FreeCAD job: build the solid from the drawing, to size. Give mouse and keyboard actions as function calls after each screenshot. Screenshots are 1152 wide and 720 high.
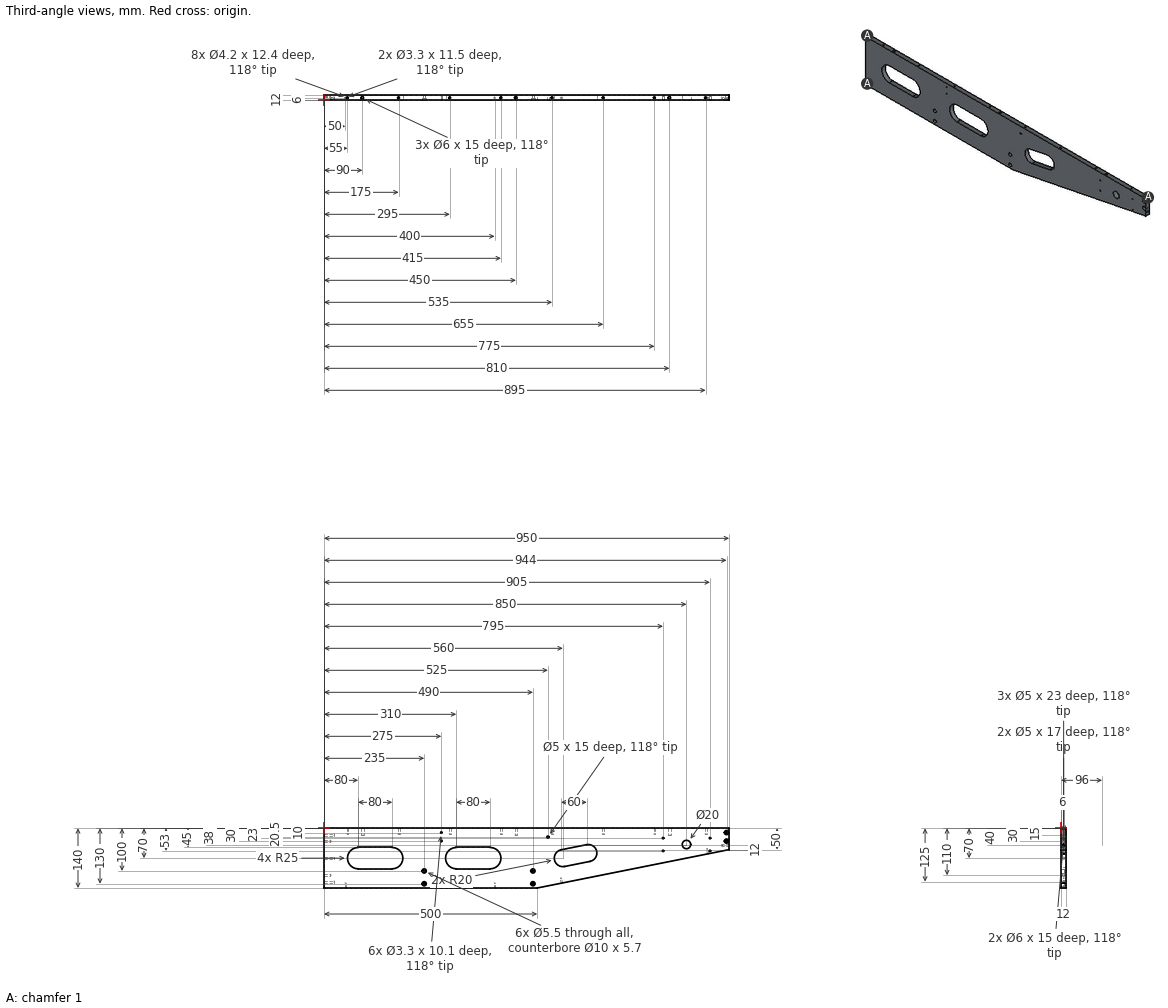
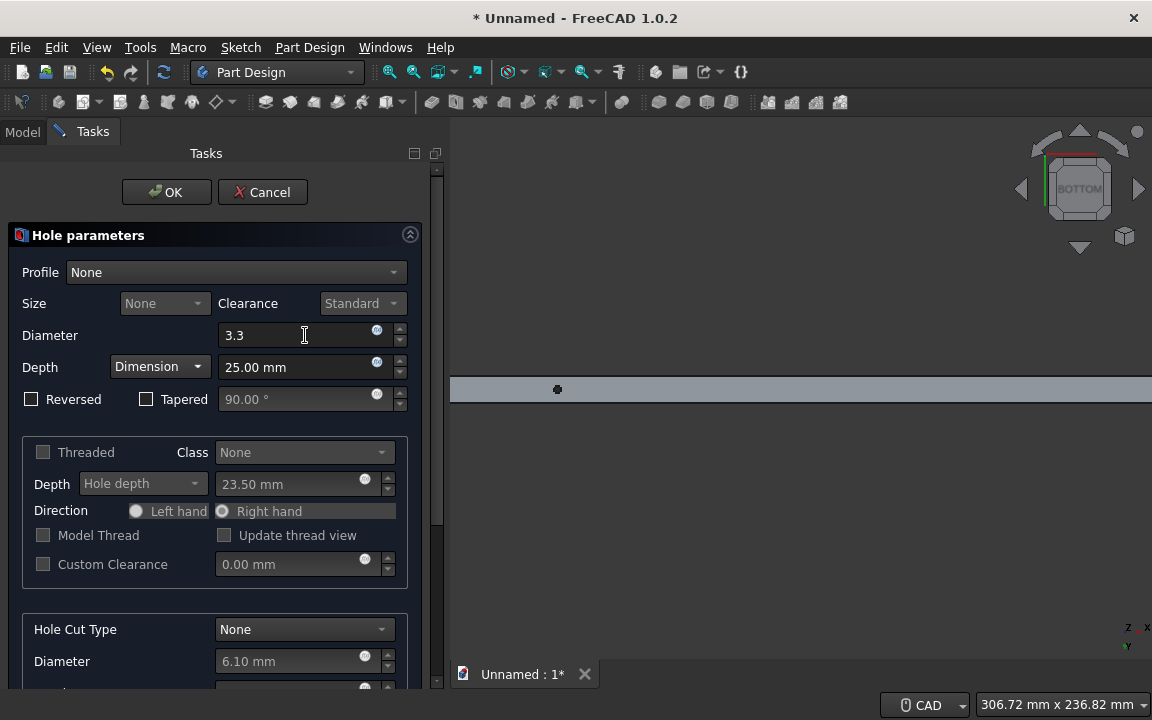
triple_click(305, 367)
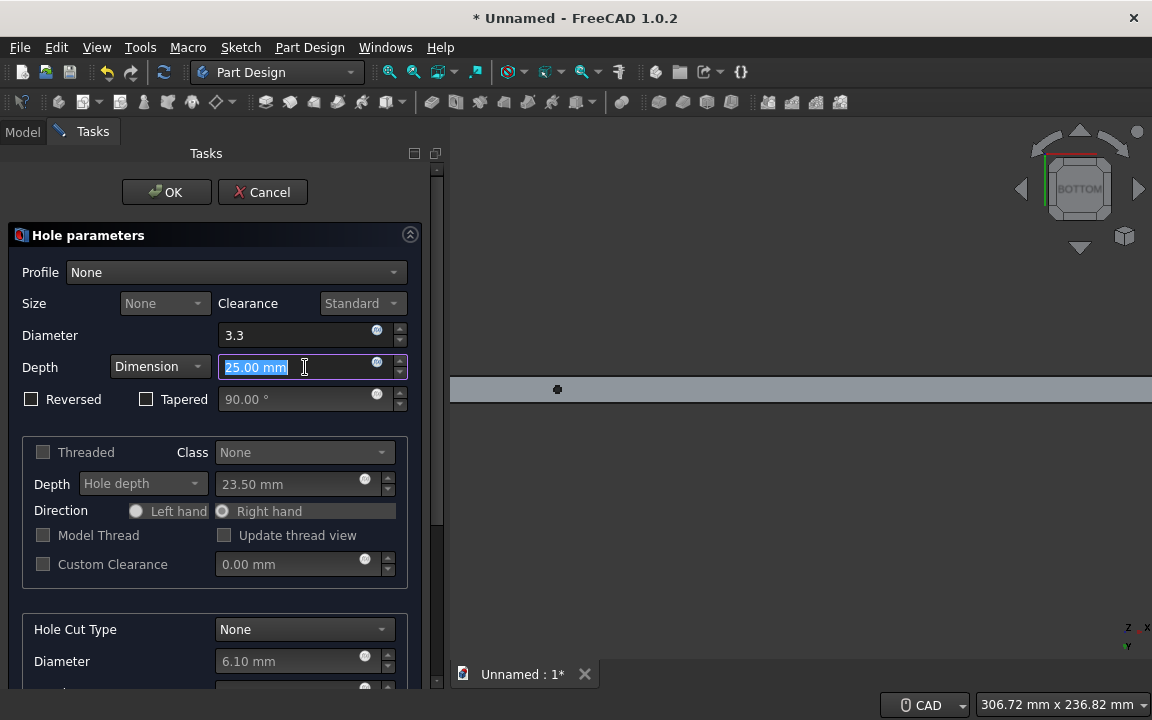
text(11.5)
key(Tab)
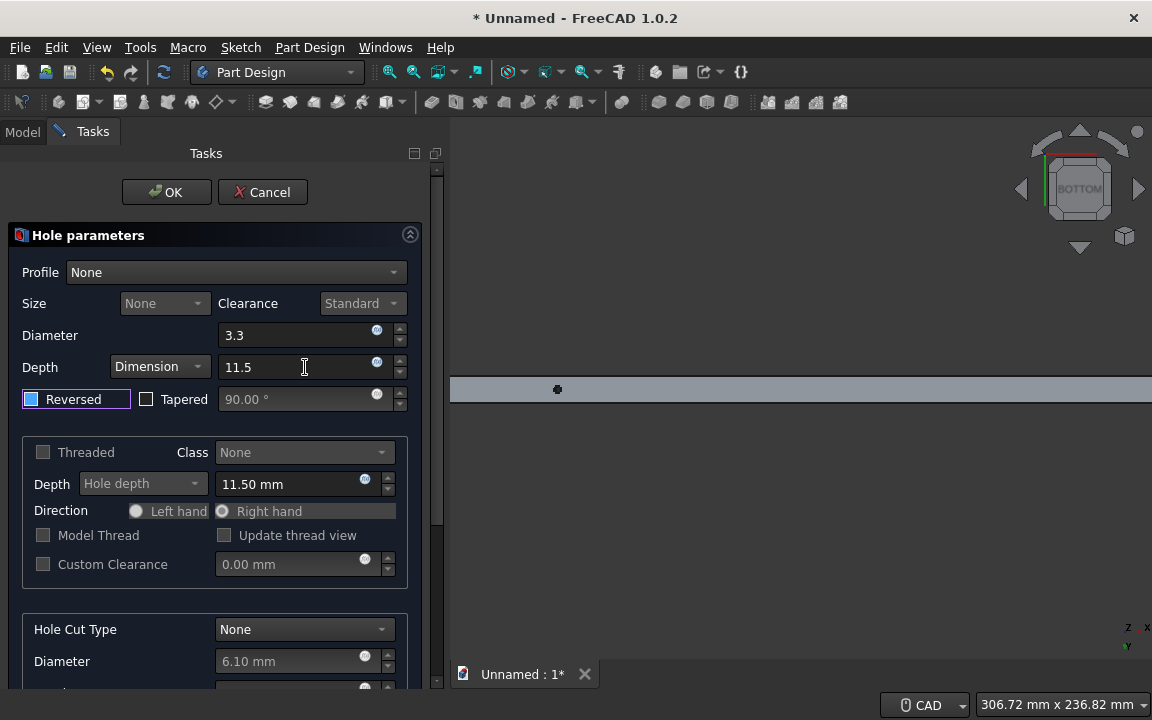
click(167, 192)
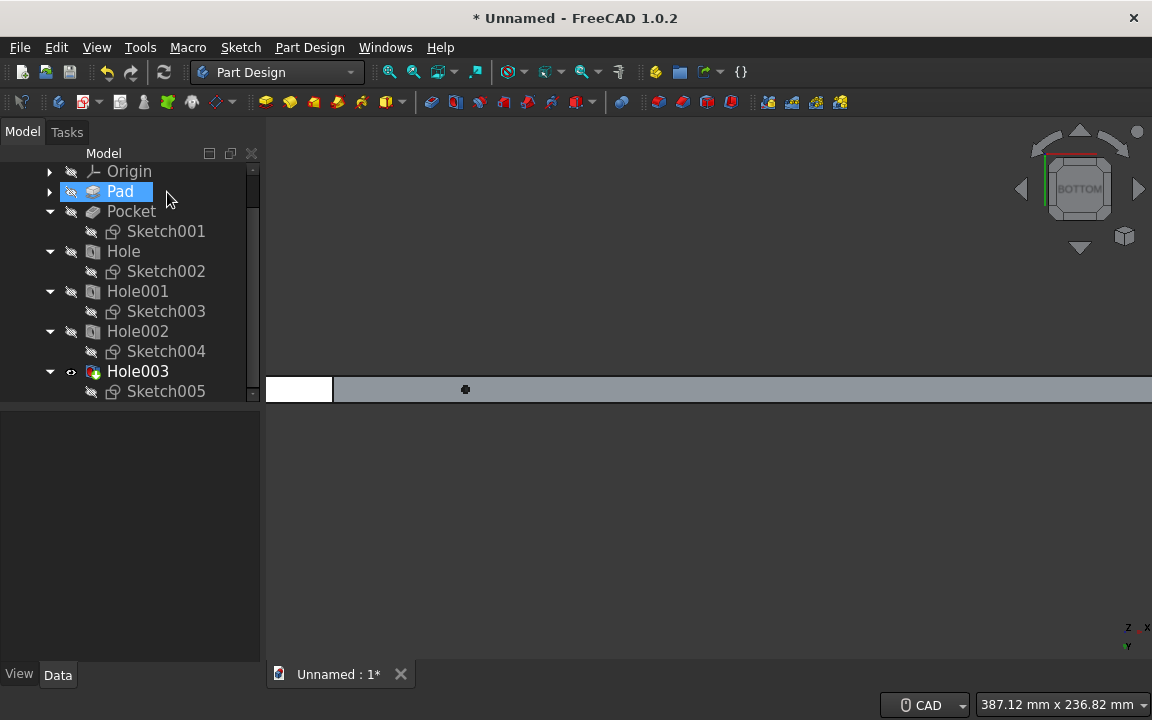
key(v)
key(f)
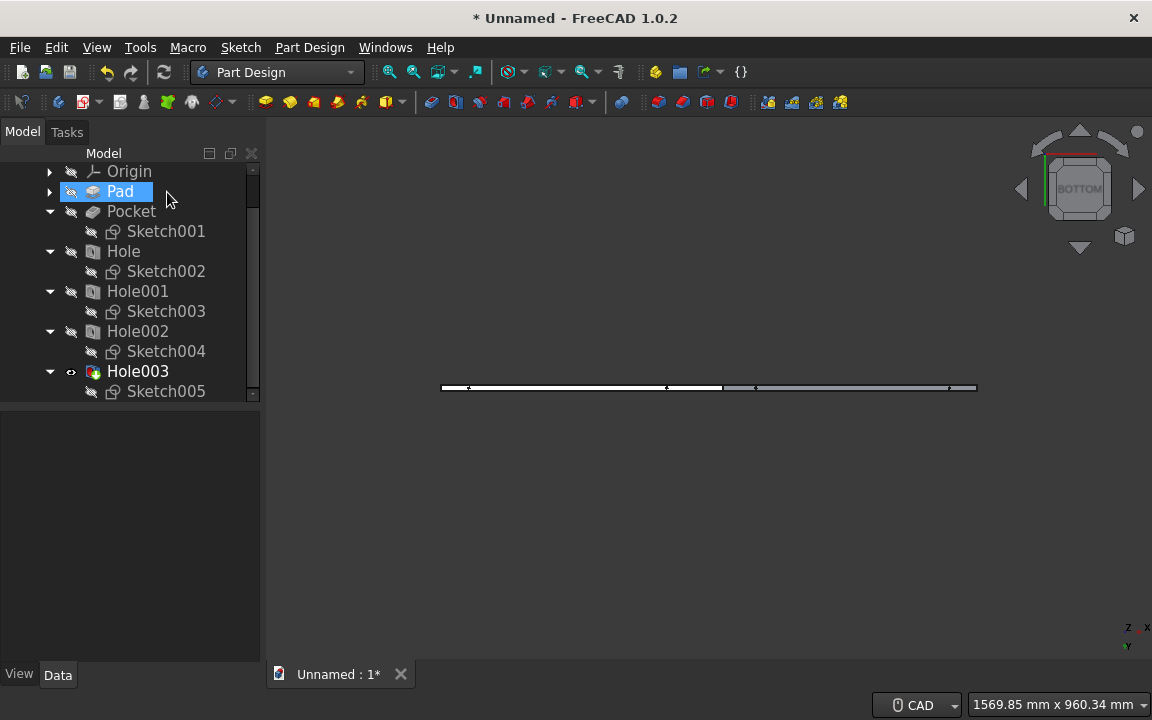
key(0)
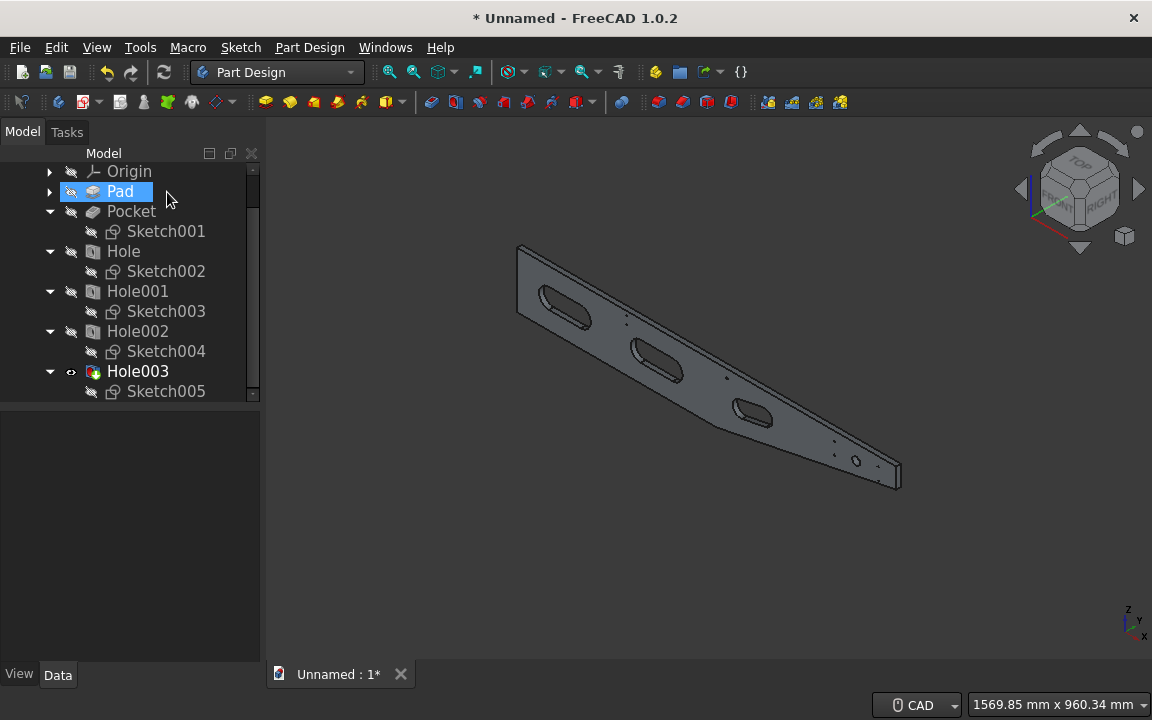
scroll(899, 469, up, 7)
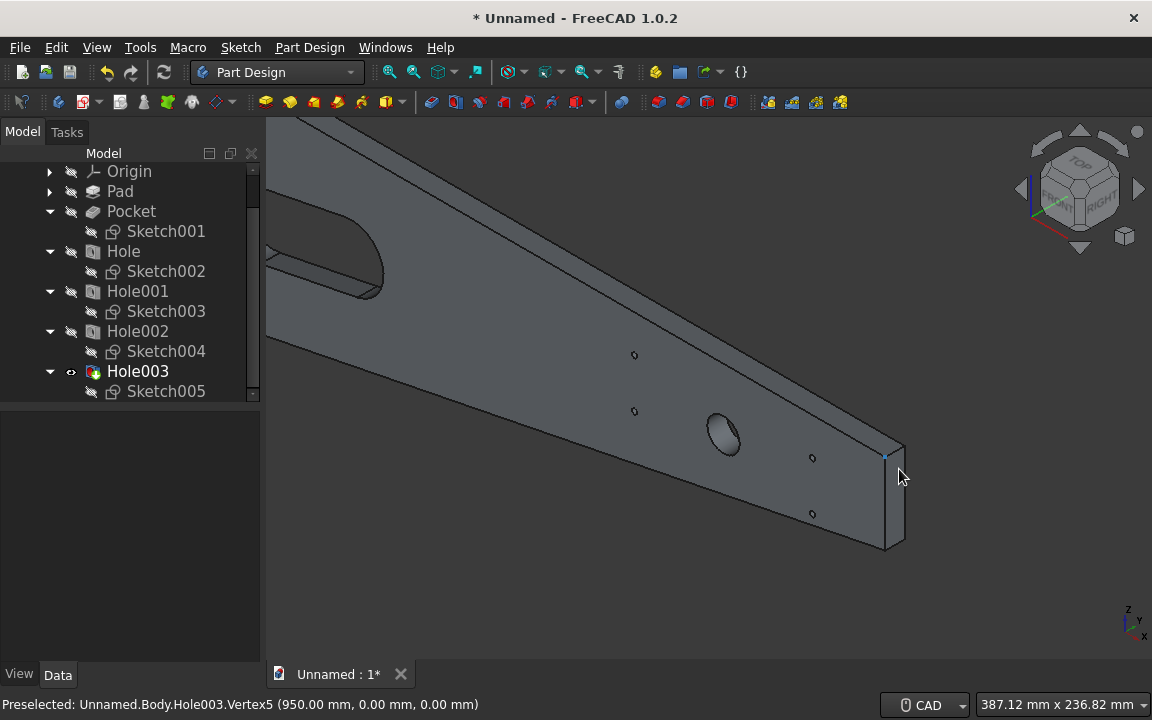
click(895, 471)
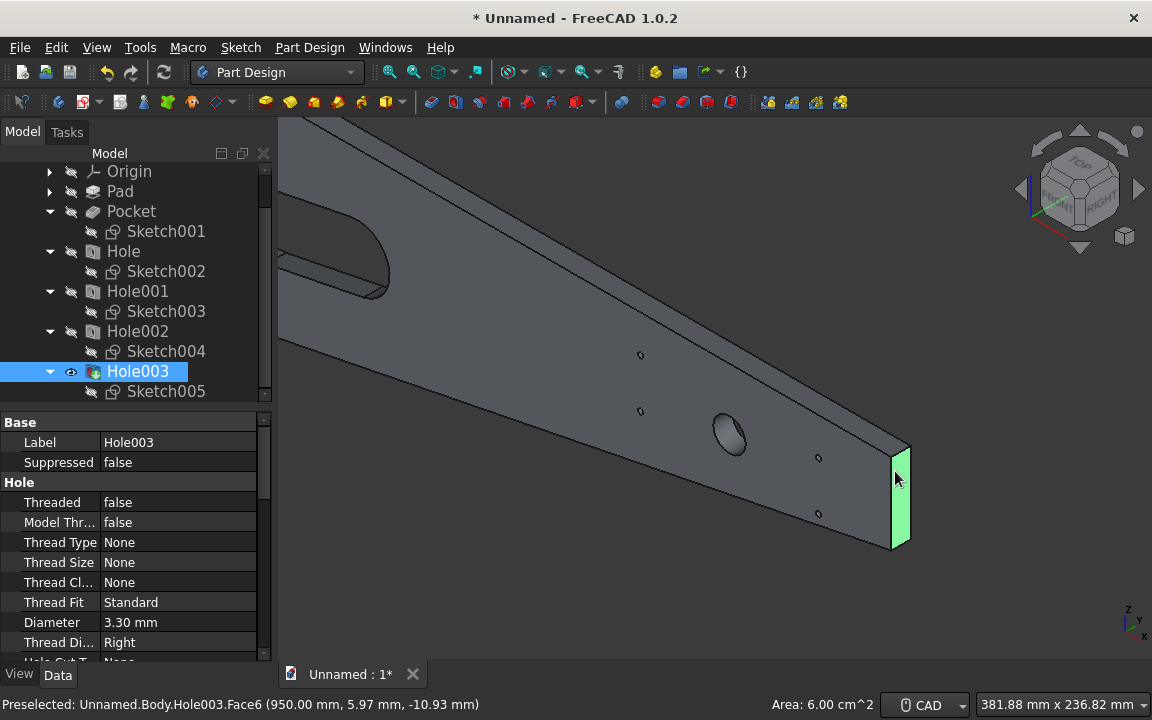
click(84, 102)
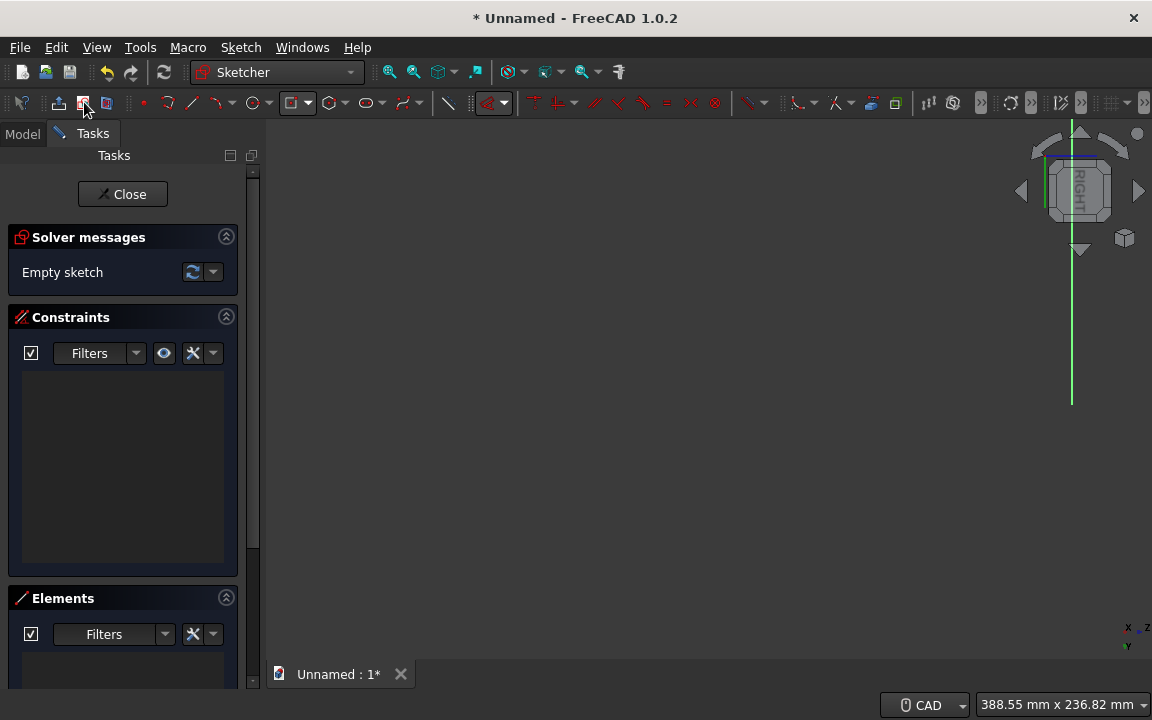
scroll(640, 389, down, 5)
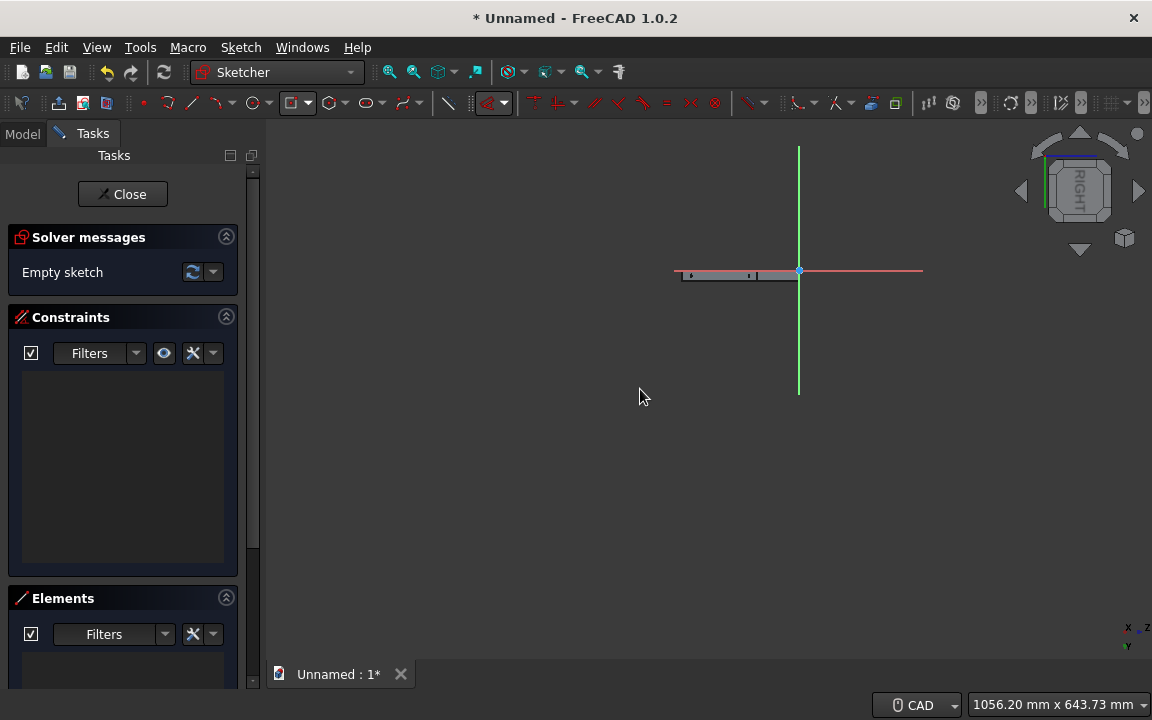
scroll(827, 287, up, 7)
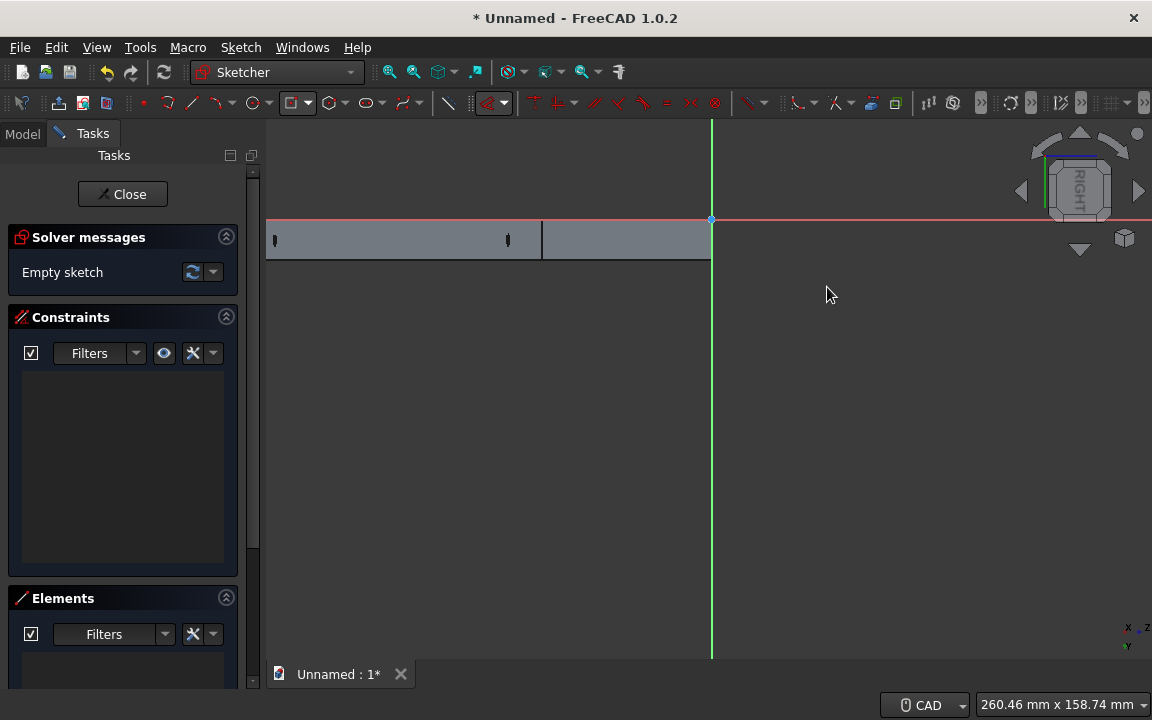
key(g)
key(c)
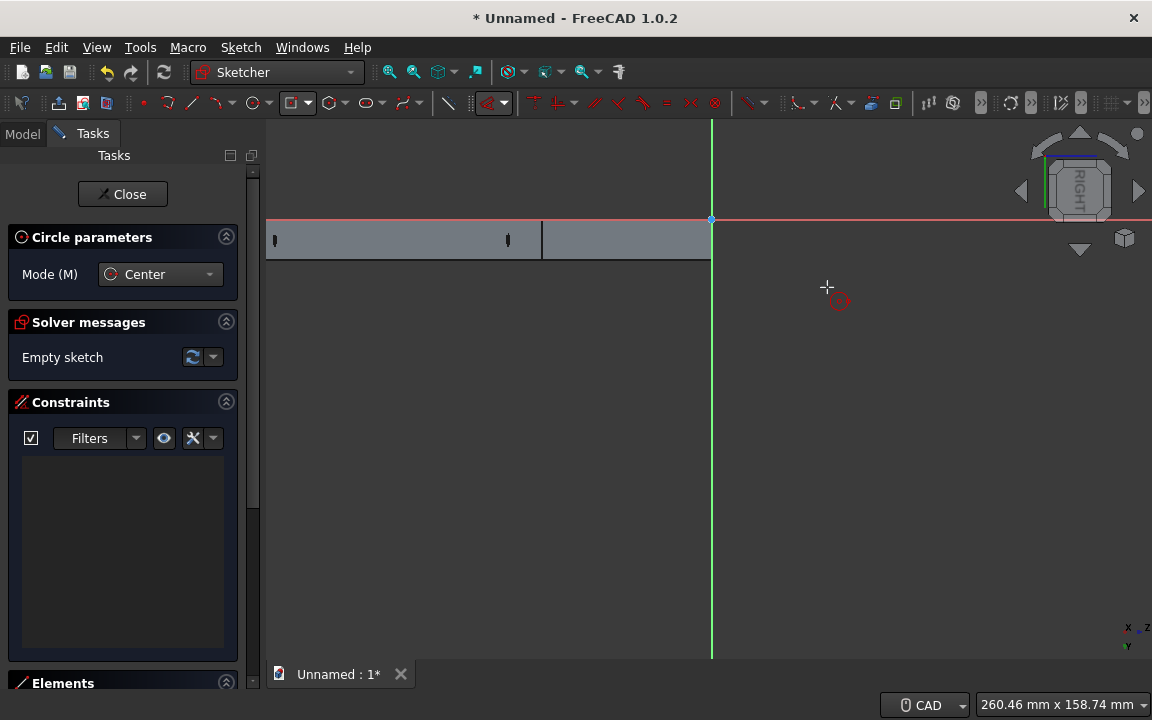
scroll(576, 240, up, 5)